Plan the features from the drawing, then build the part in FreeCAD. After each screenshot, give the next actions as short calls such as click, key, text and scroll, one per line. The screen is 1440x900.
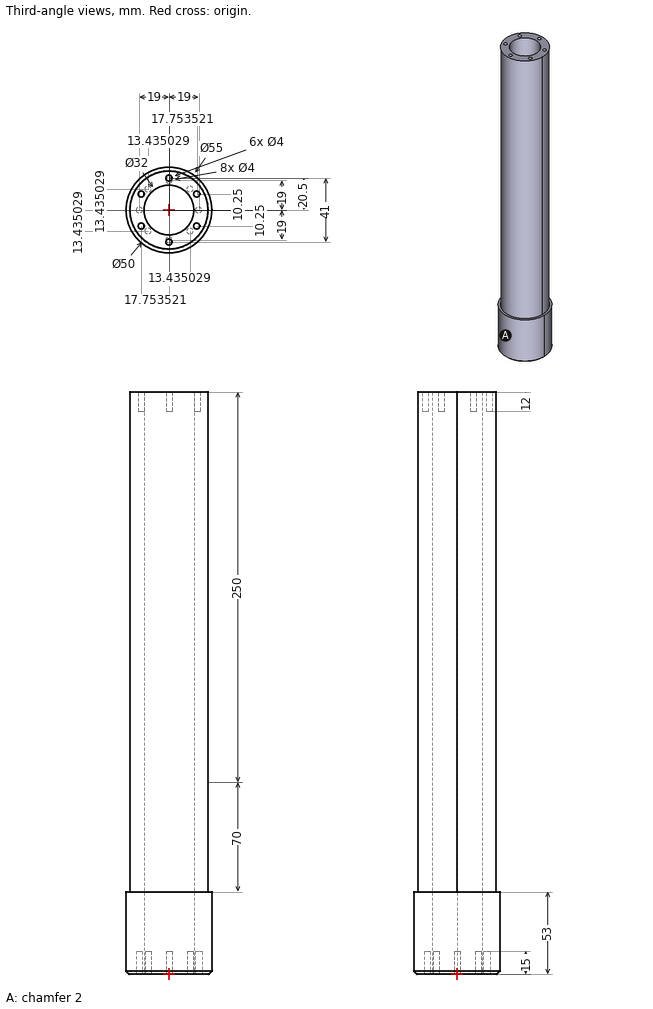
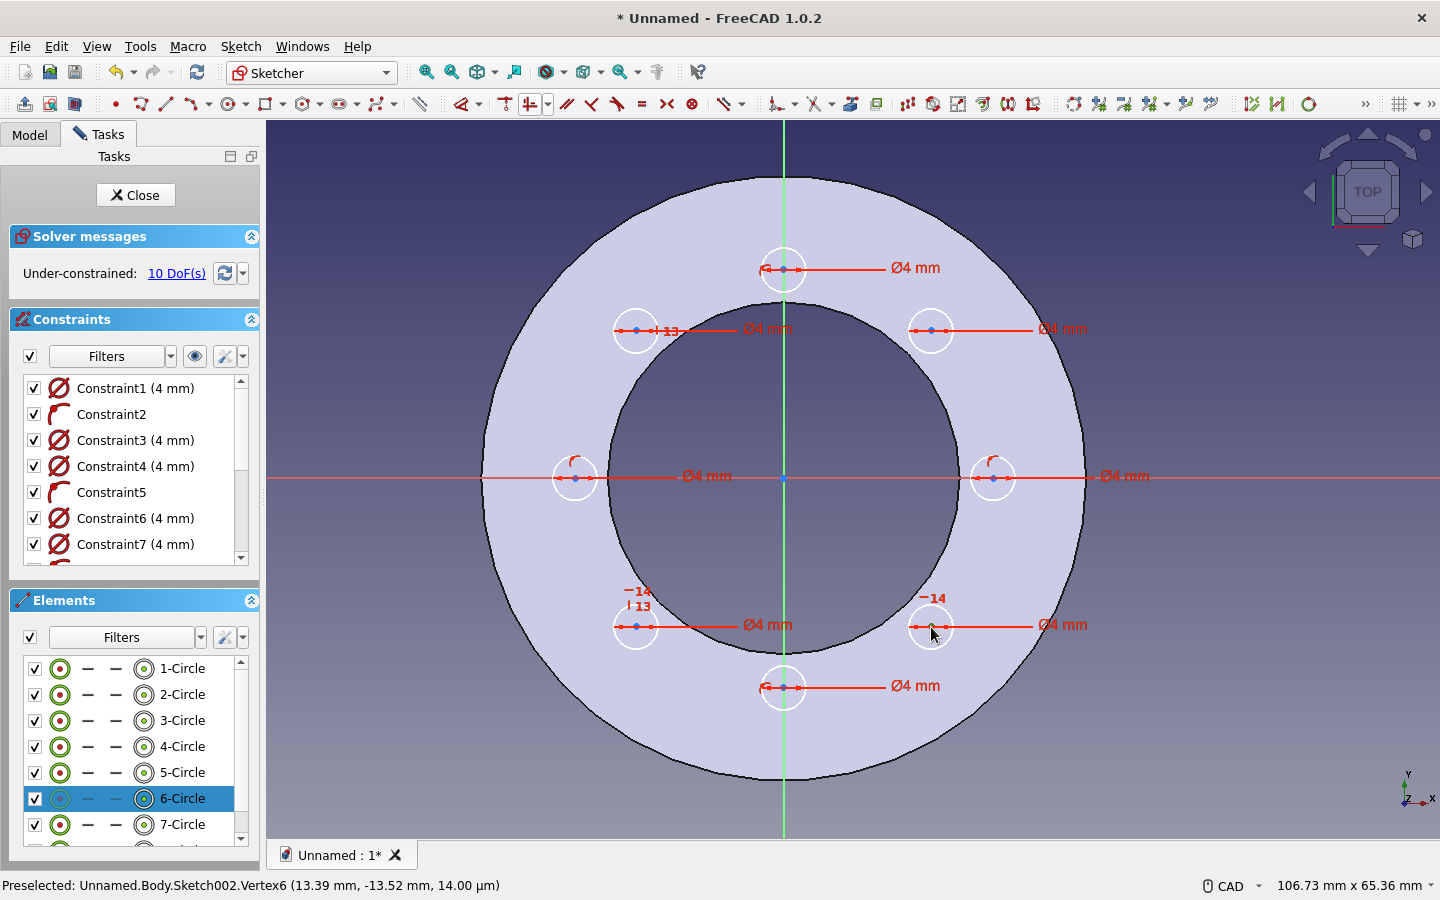
click(931, 331)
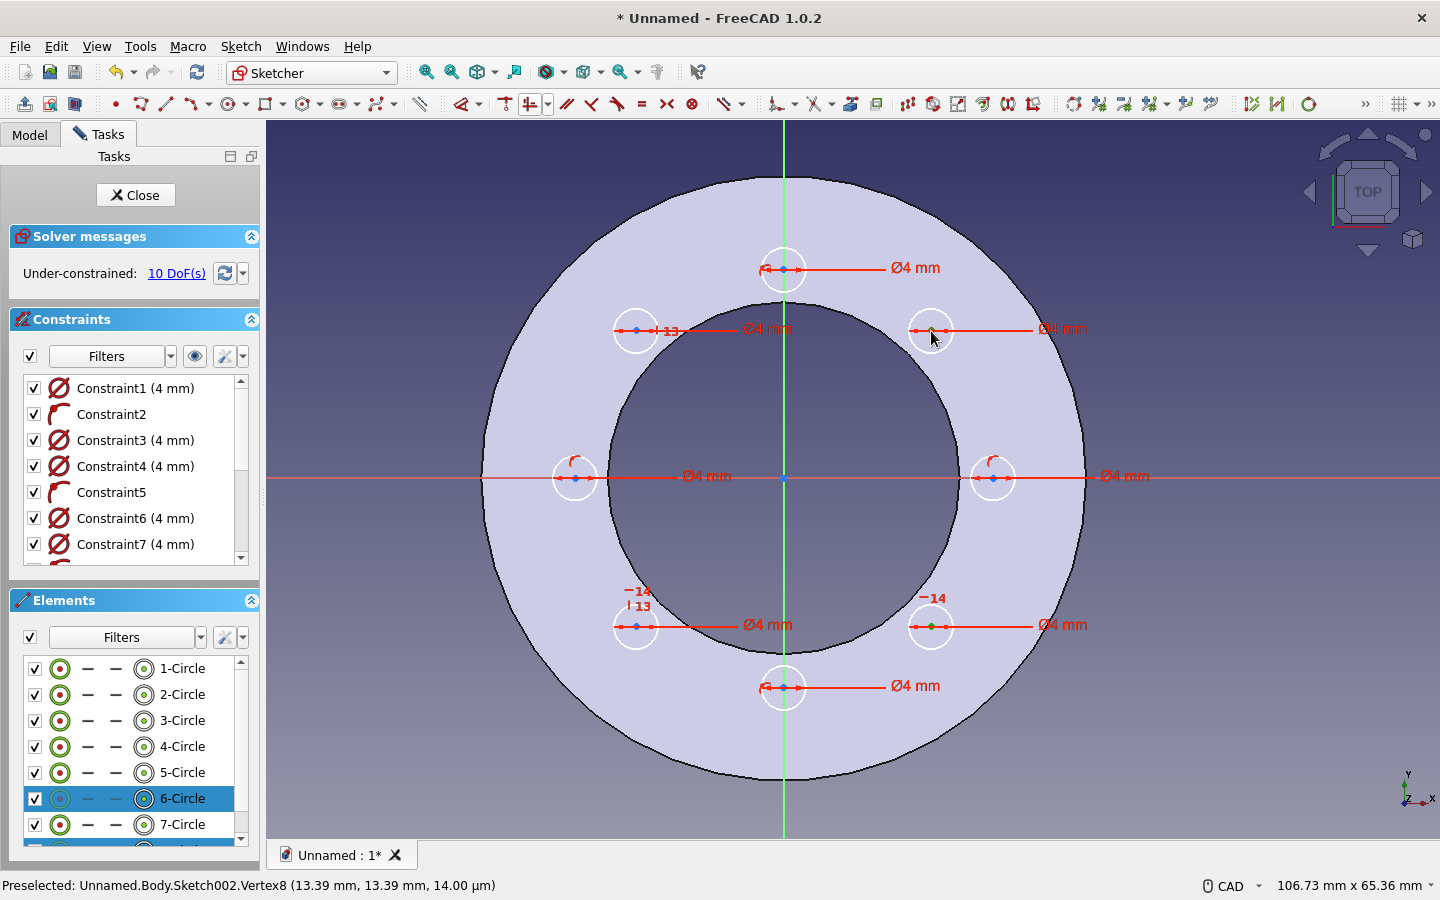
click(548, 104)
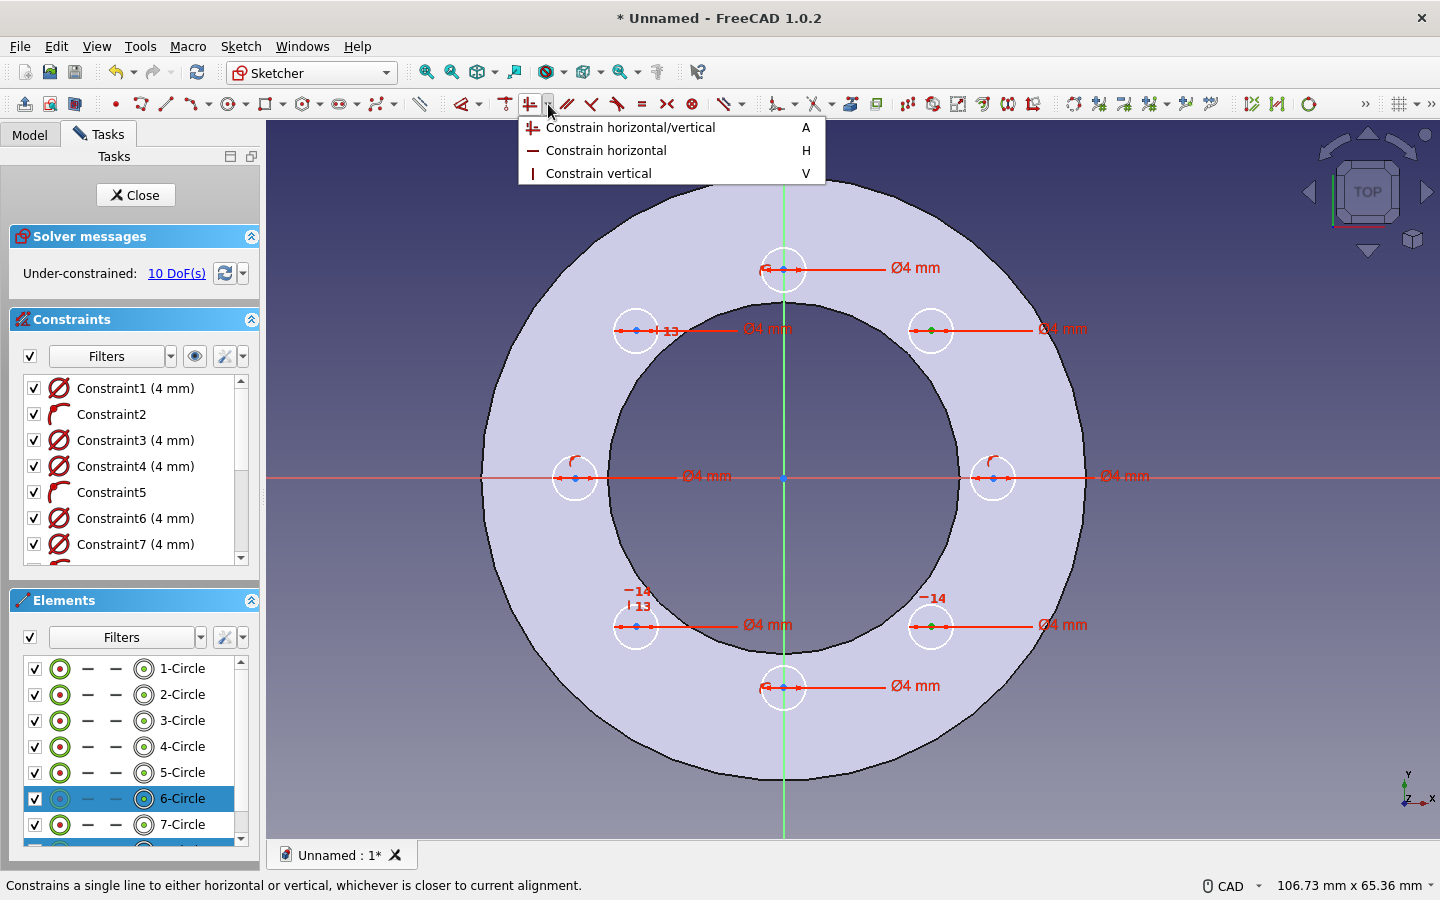
click(672, 174)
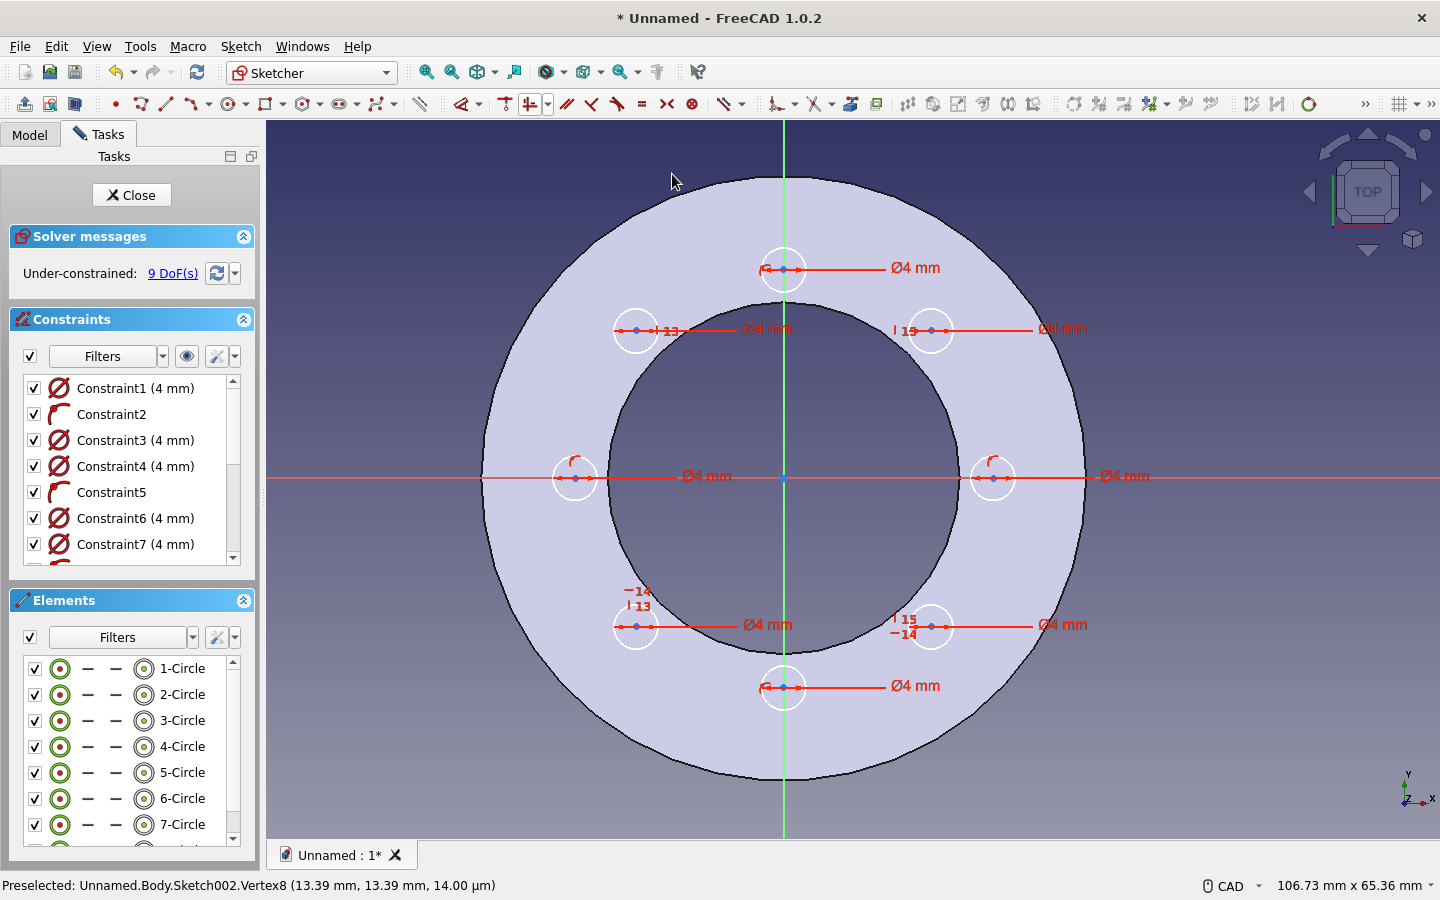
click(636, 331)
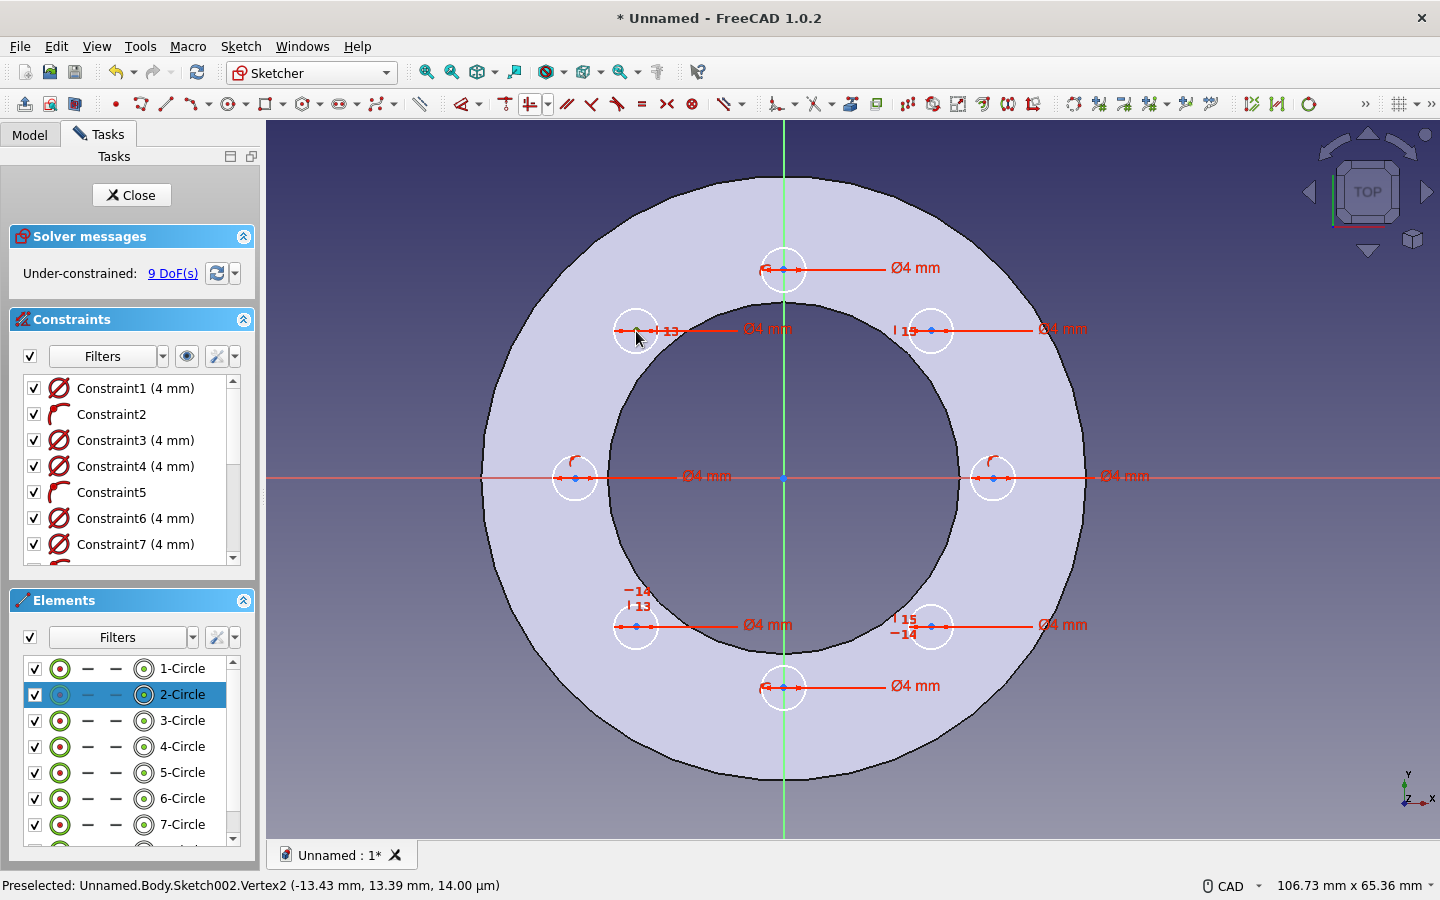
click(931, 331)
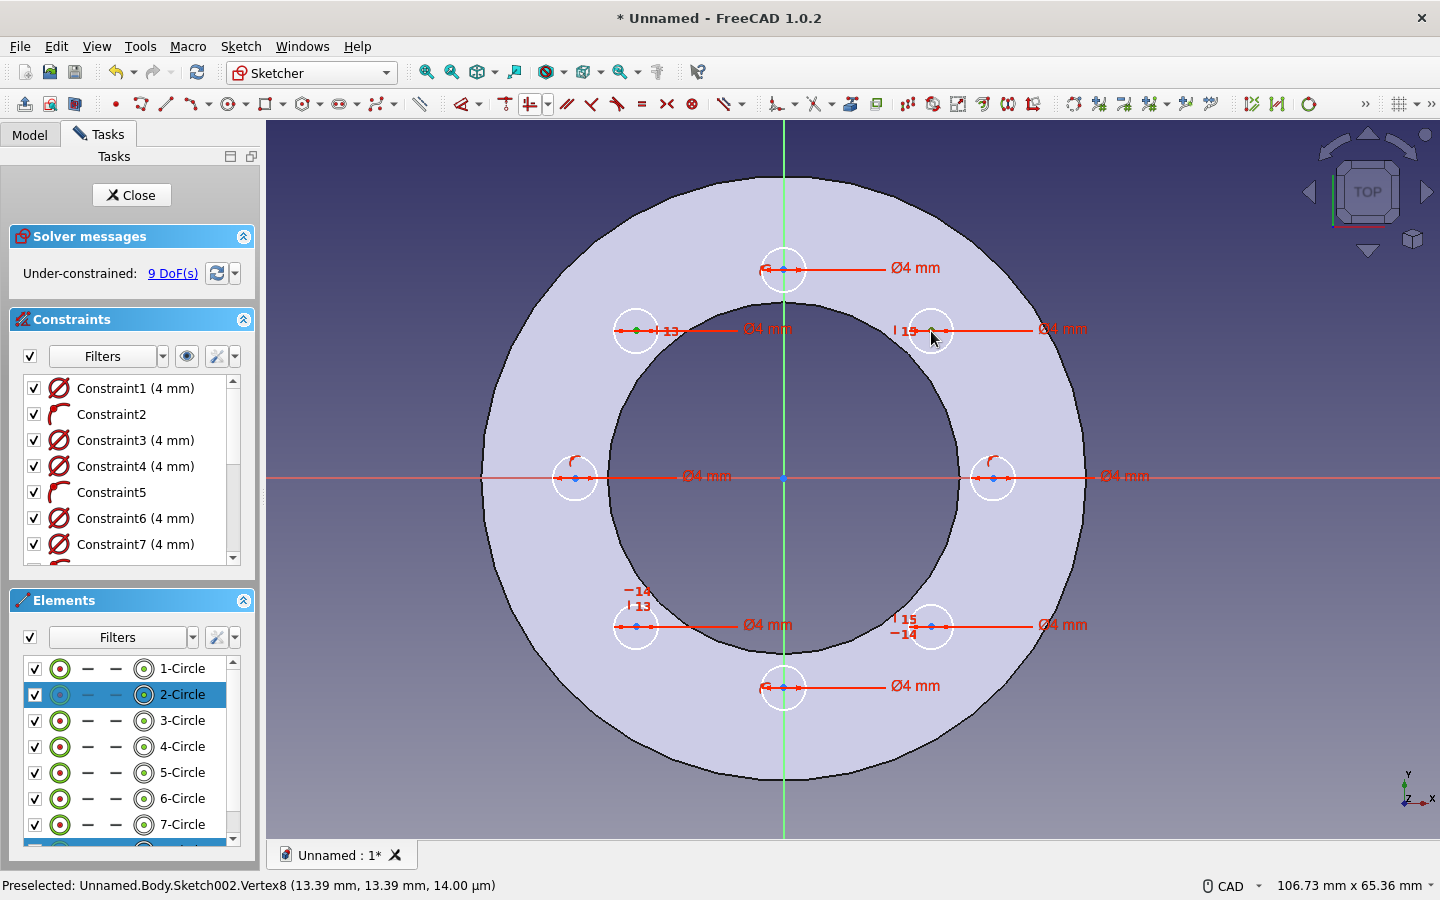
click(548, 104)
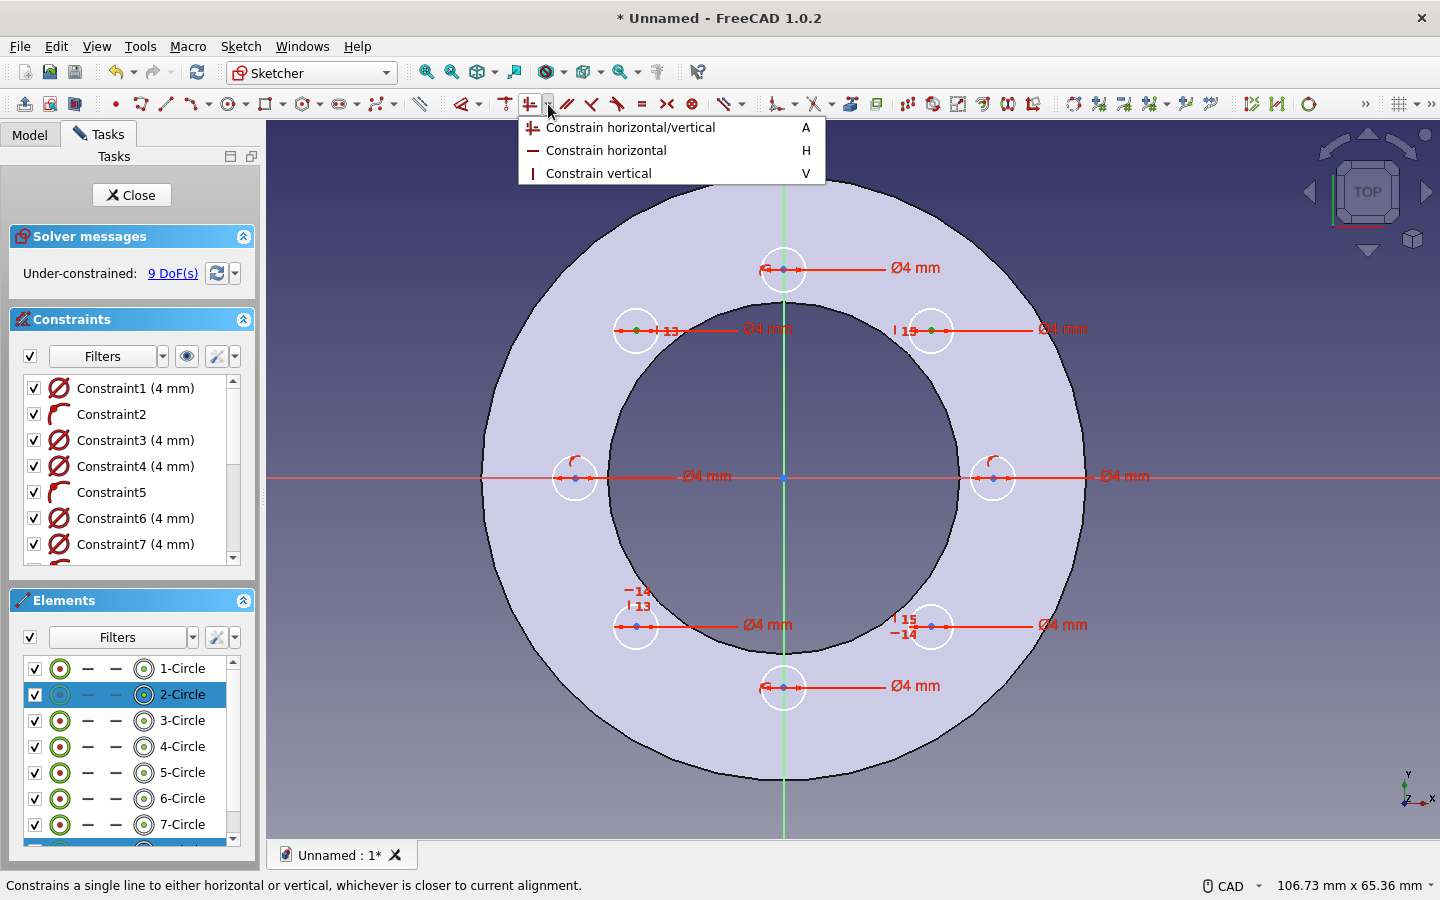
click(672, 150)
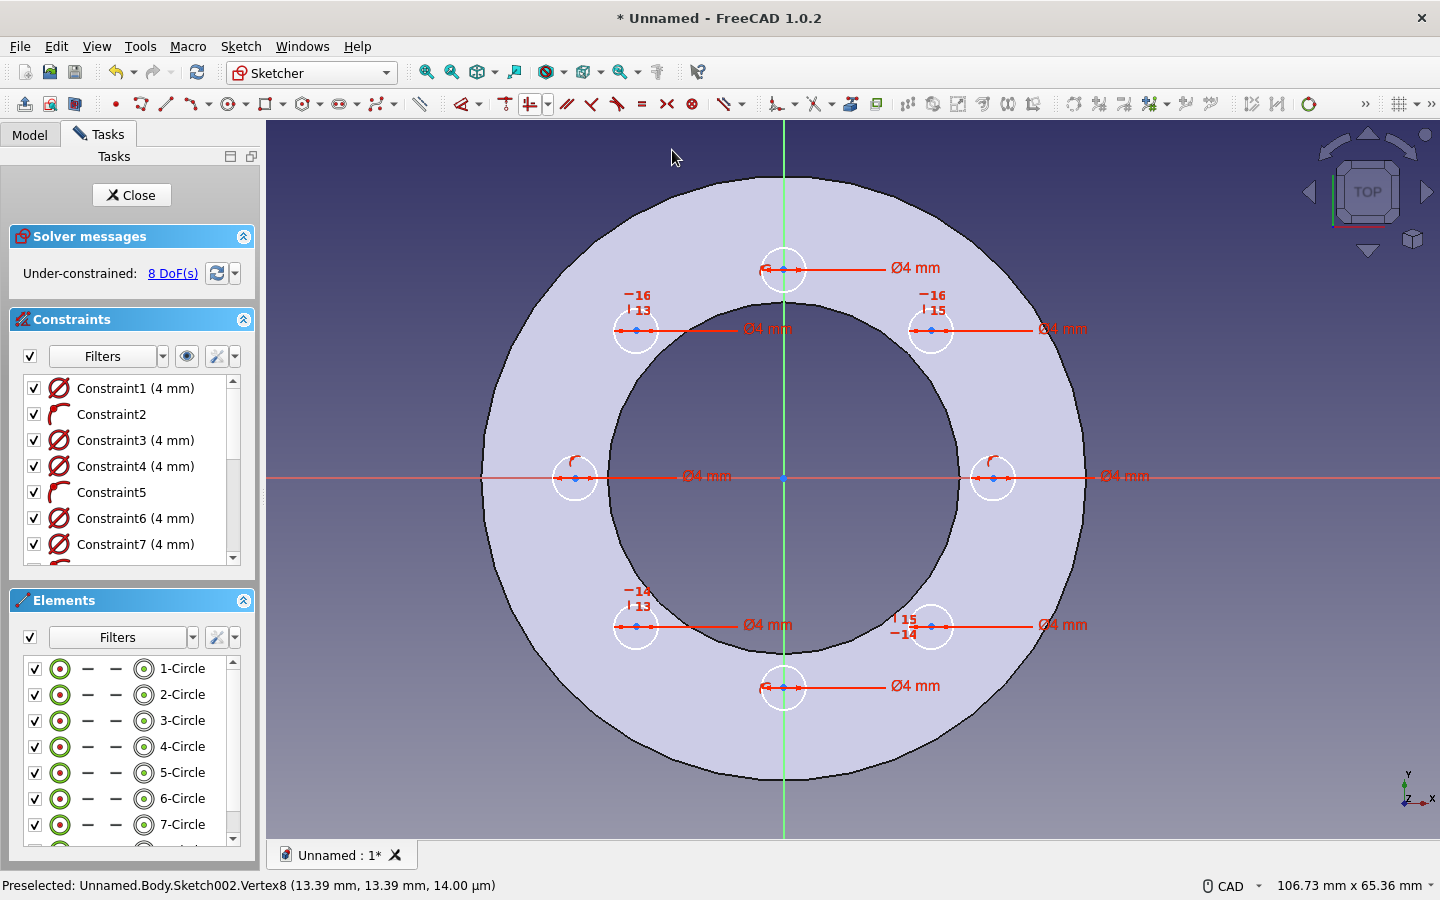
click(460, 104)